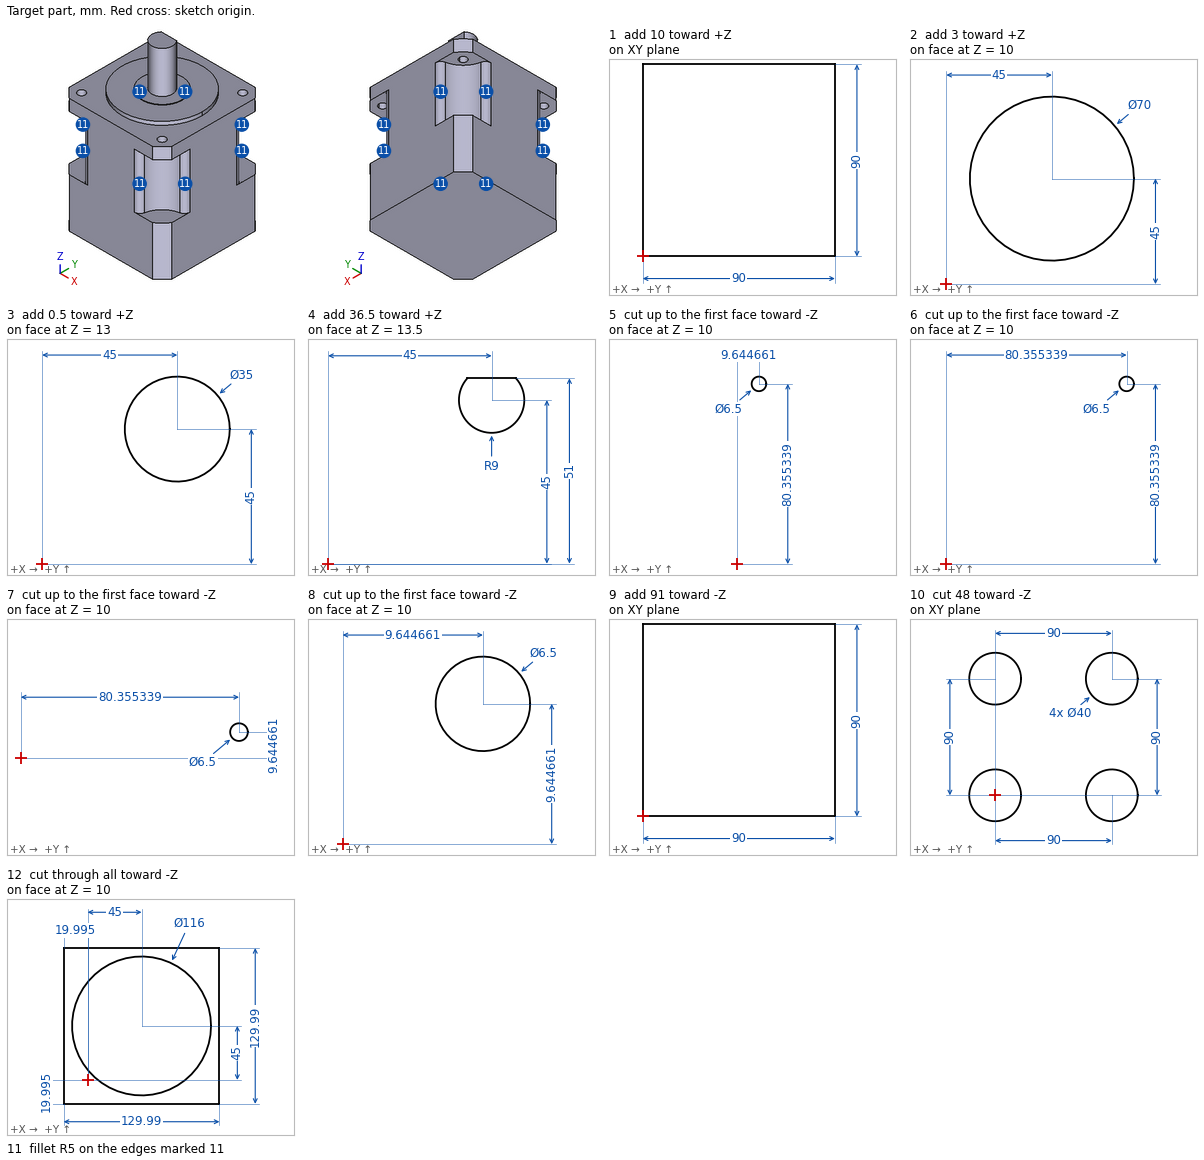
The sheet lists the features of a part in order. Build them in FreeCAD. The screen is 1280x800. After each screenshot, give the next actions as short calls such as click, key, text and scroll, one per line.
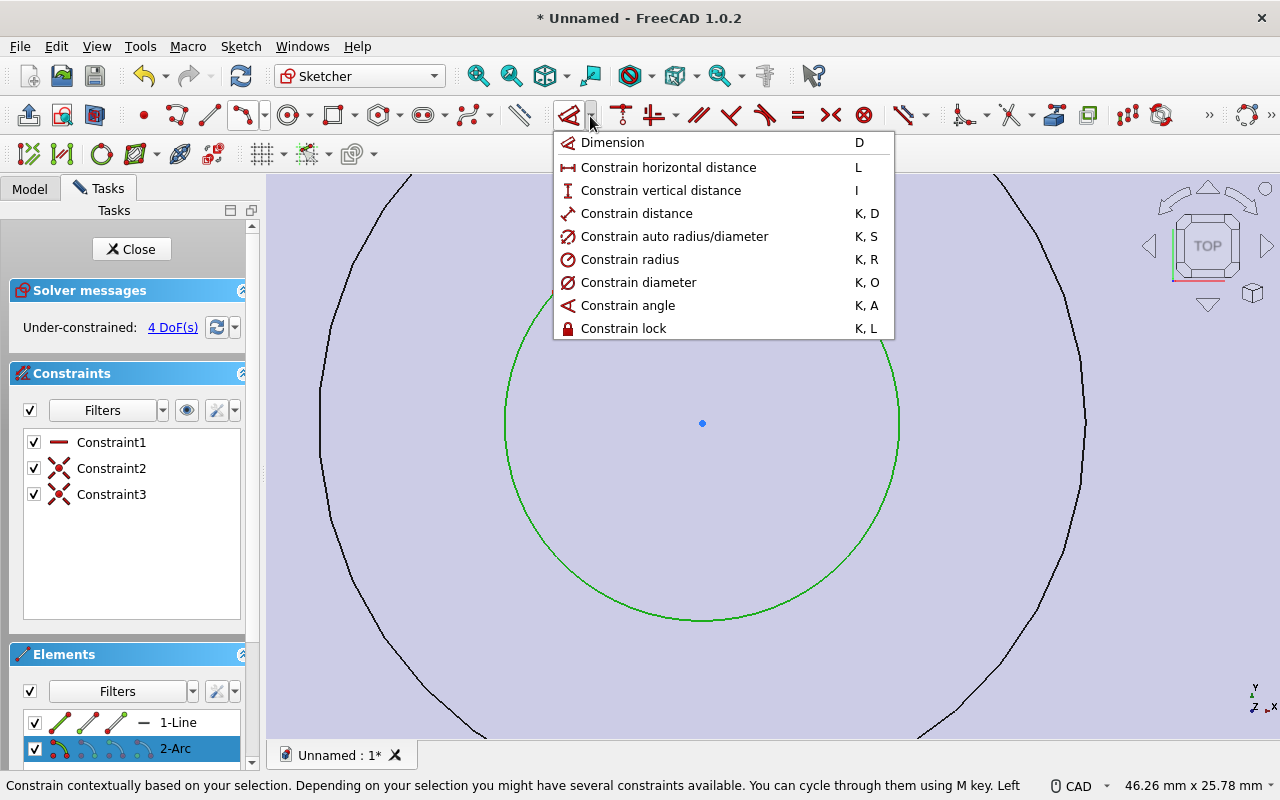
click(724, 260)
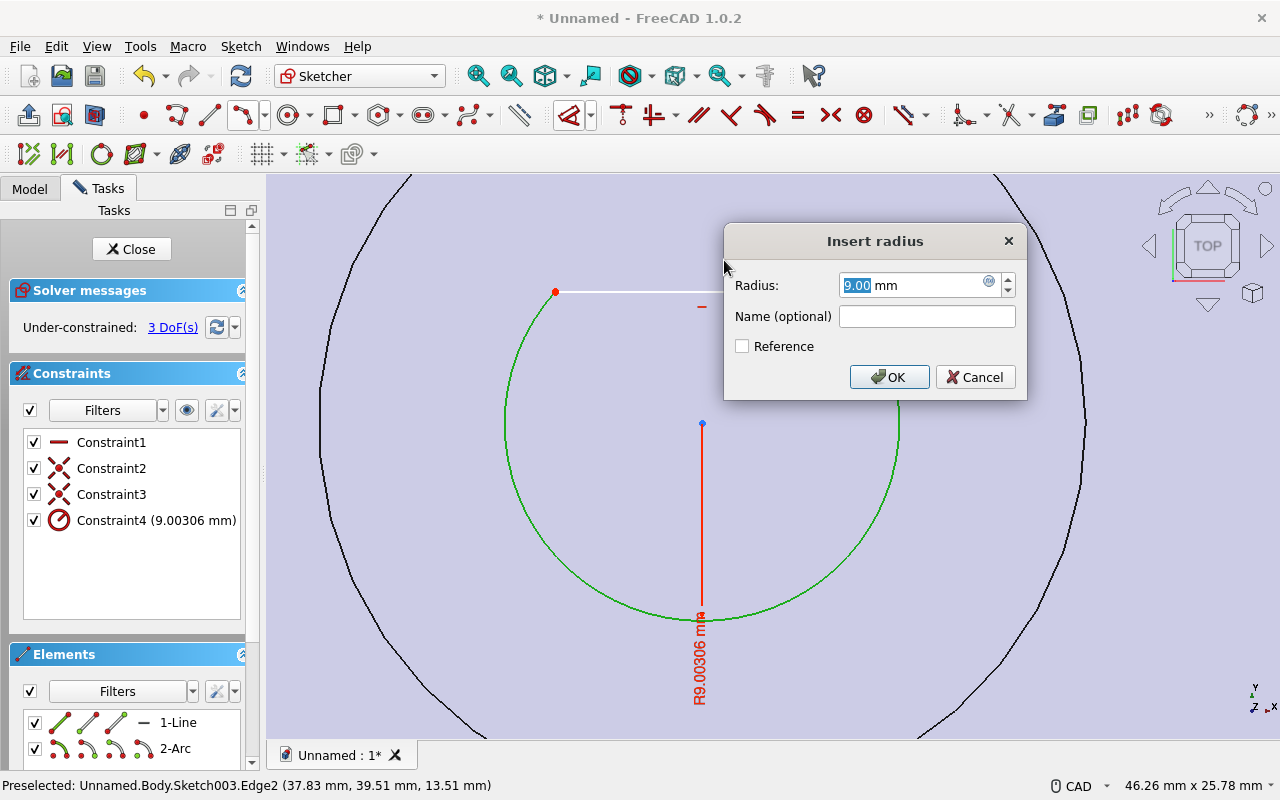
text(9)
key(Return)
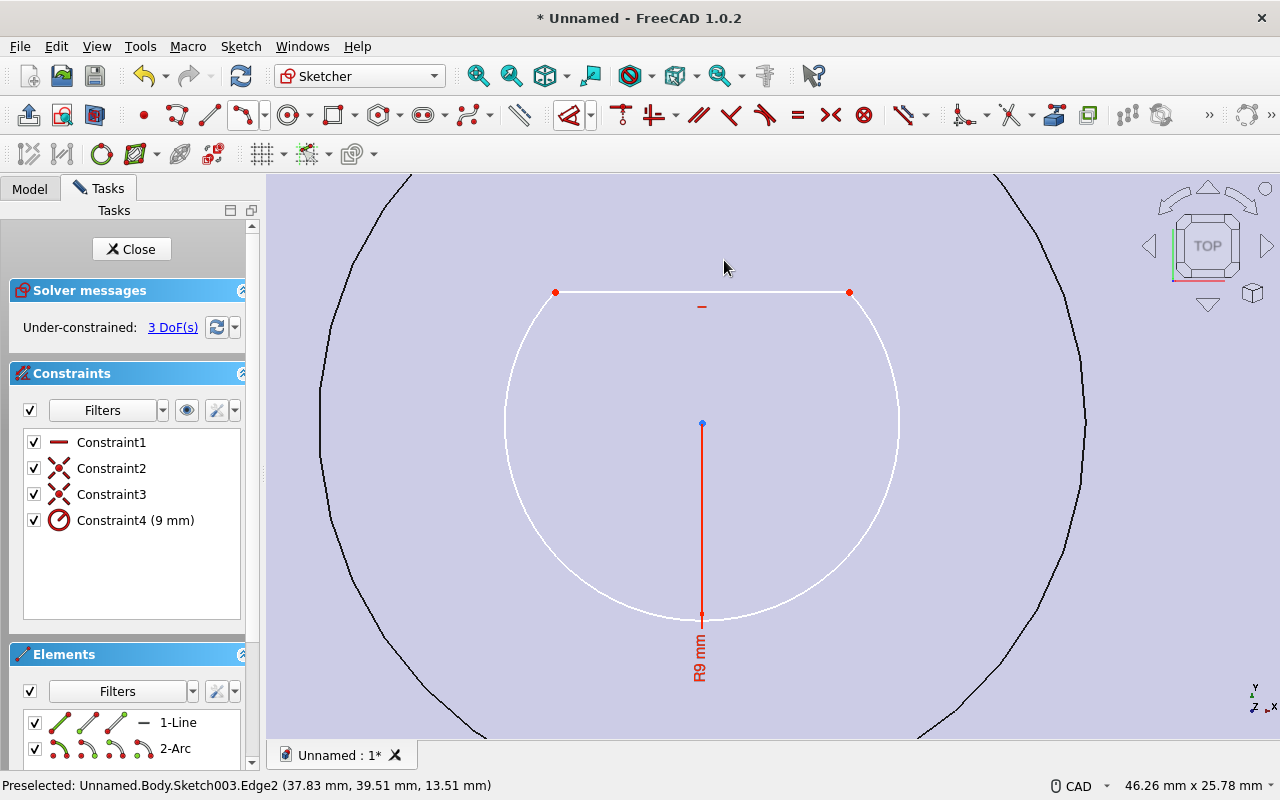
click(849, 292)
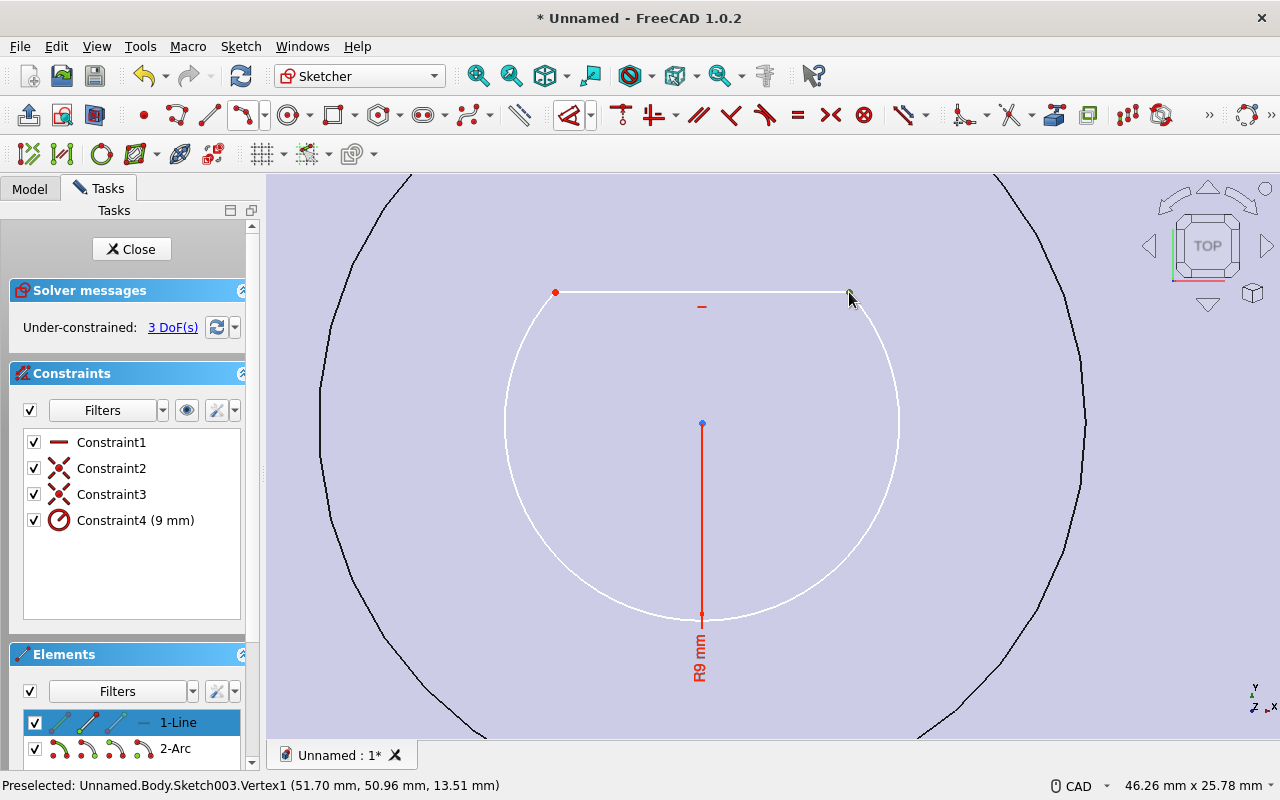
key(i)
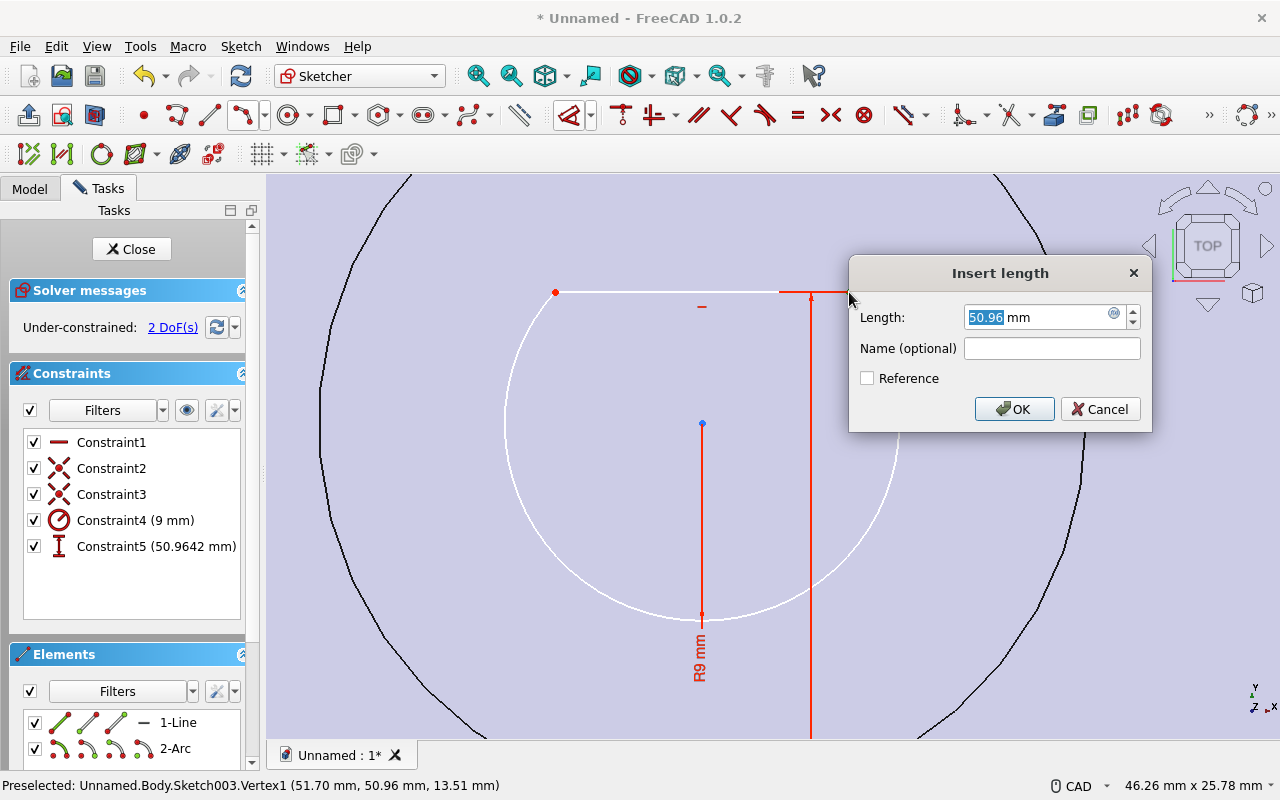
text(51)
key(Return)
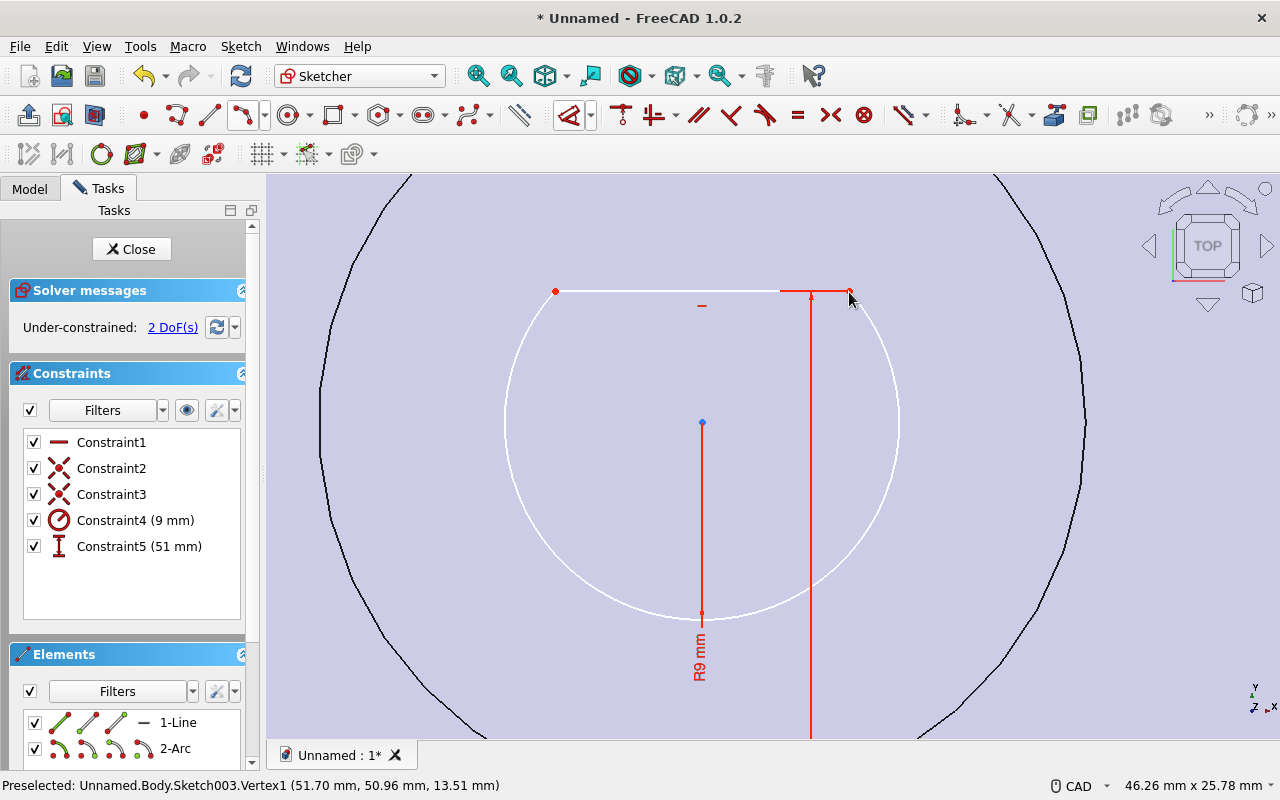
click(702, 423)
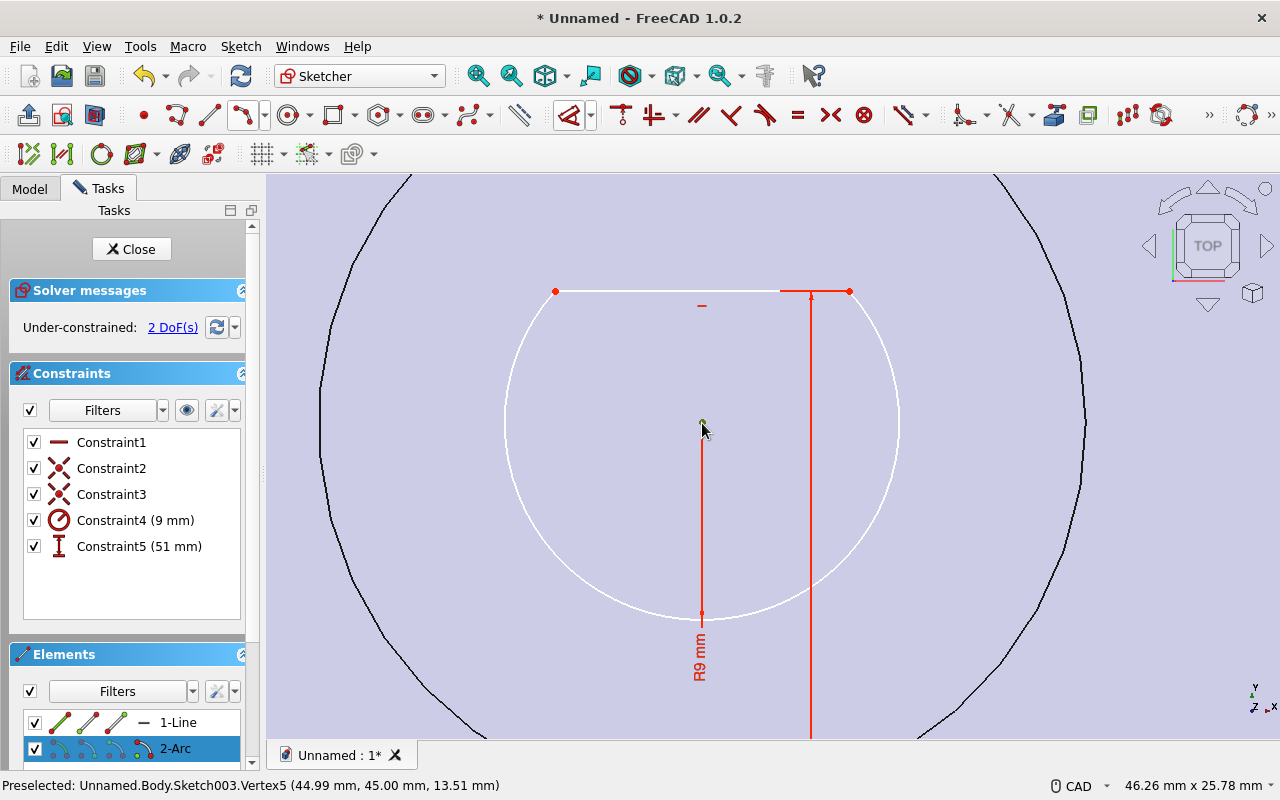
key(l)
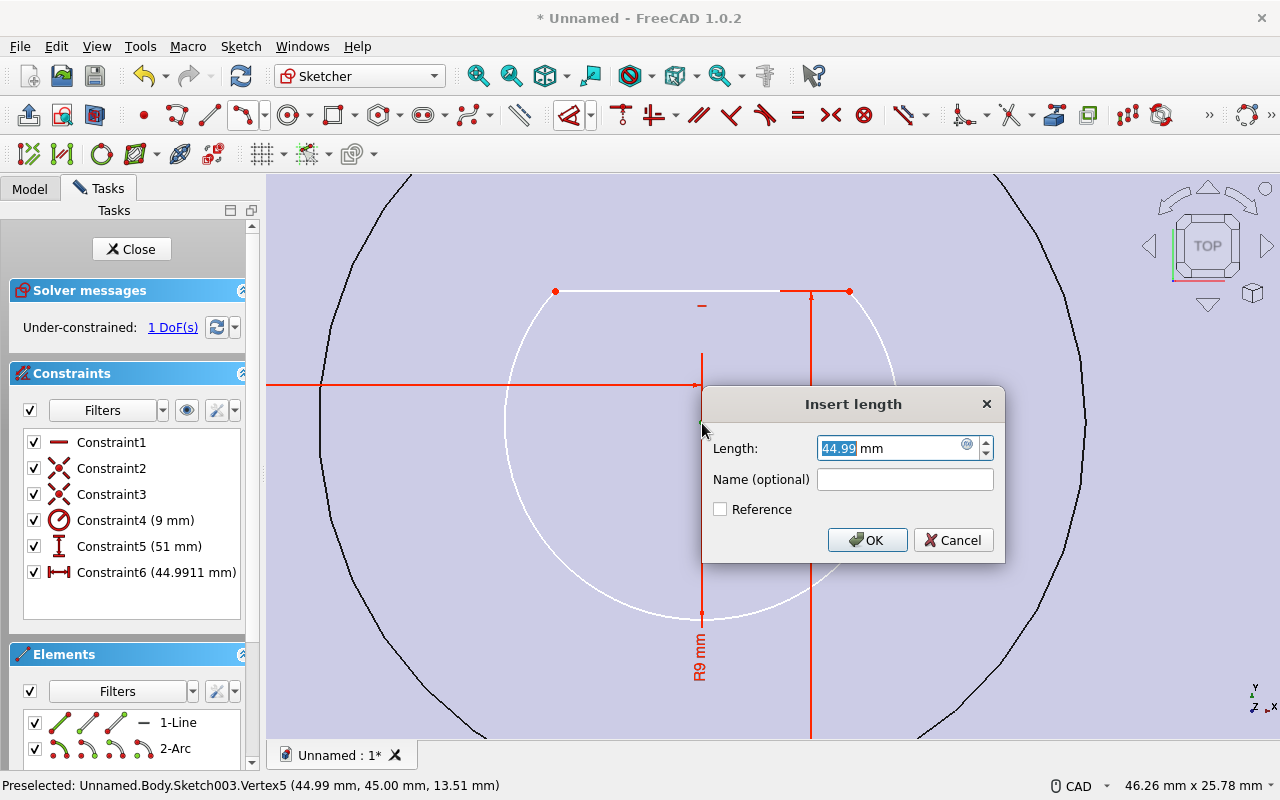
text(45)
key(Return)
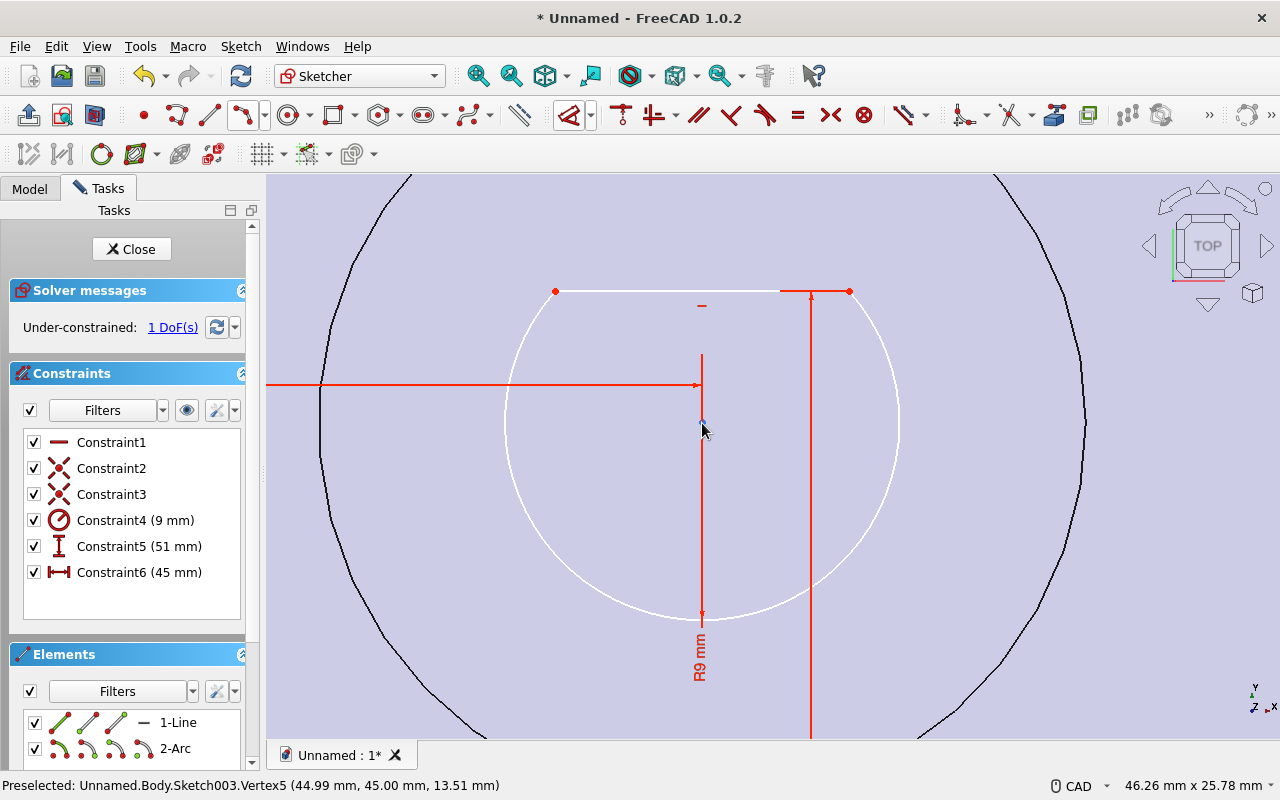
click(702, 423)